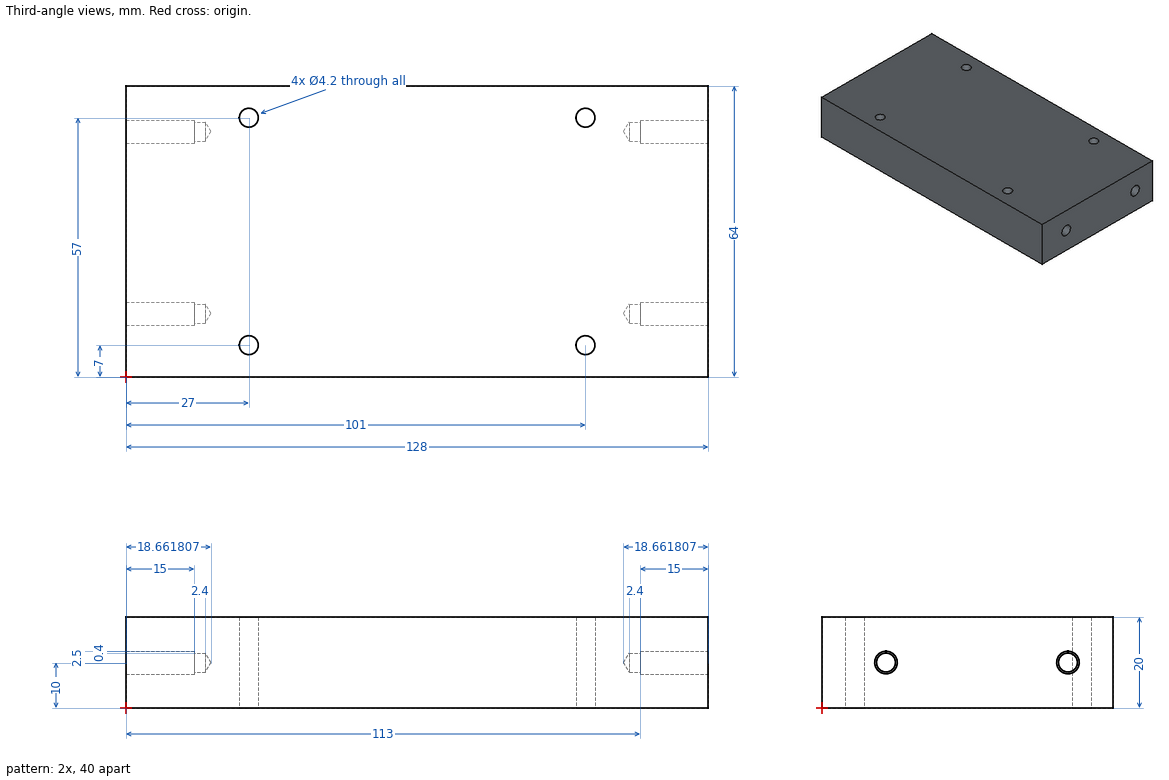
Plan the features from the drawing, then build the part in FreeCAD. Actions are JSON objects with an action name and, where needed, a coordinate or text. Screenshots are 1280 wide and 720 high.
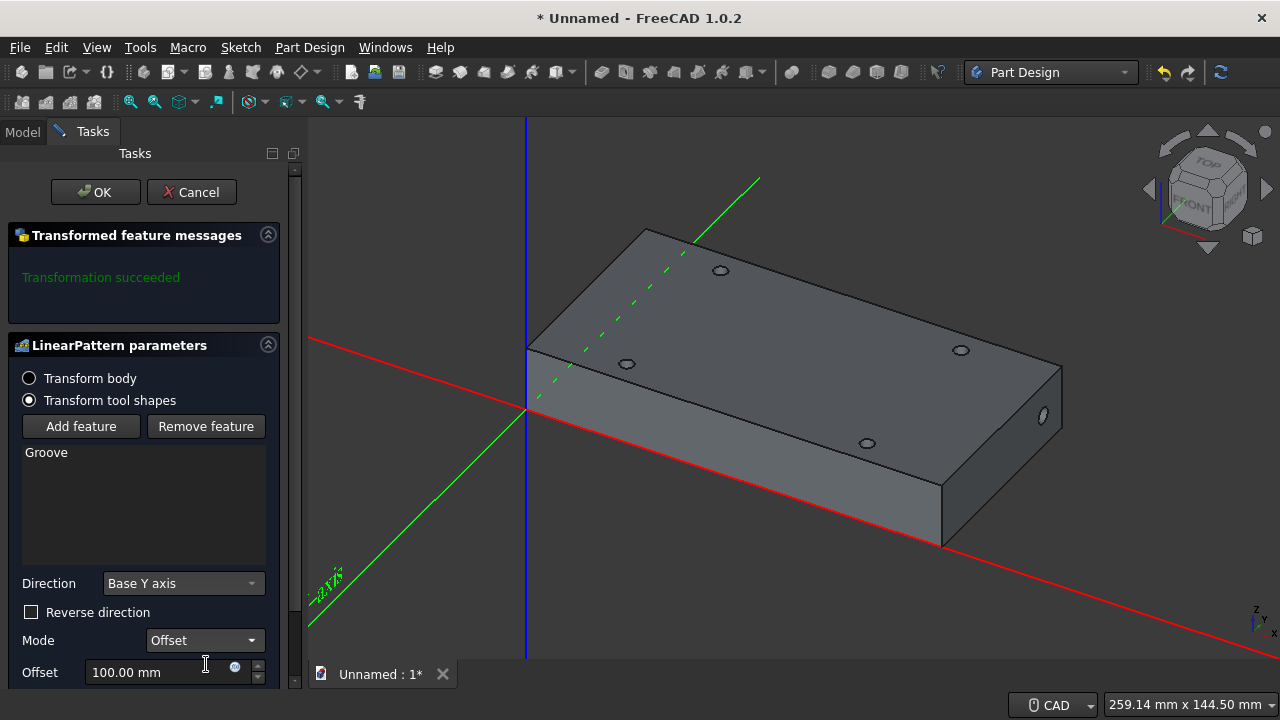
{"action": "triple_click", "coordinate": [168, 672]}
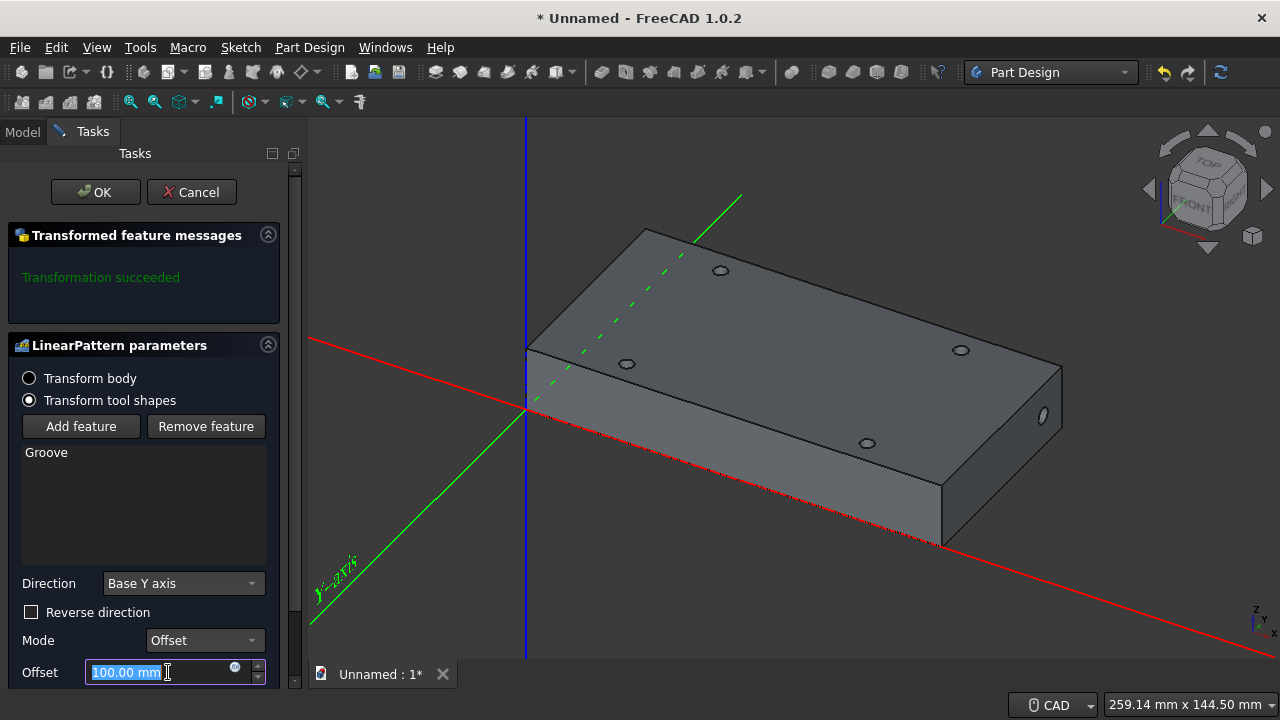
{"action": "type", "text": "40"}
{"action": "key", "text": "Tab"}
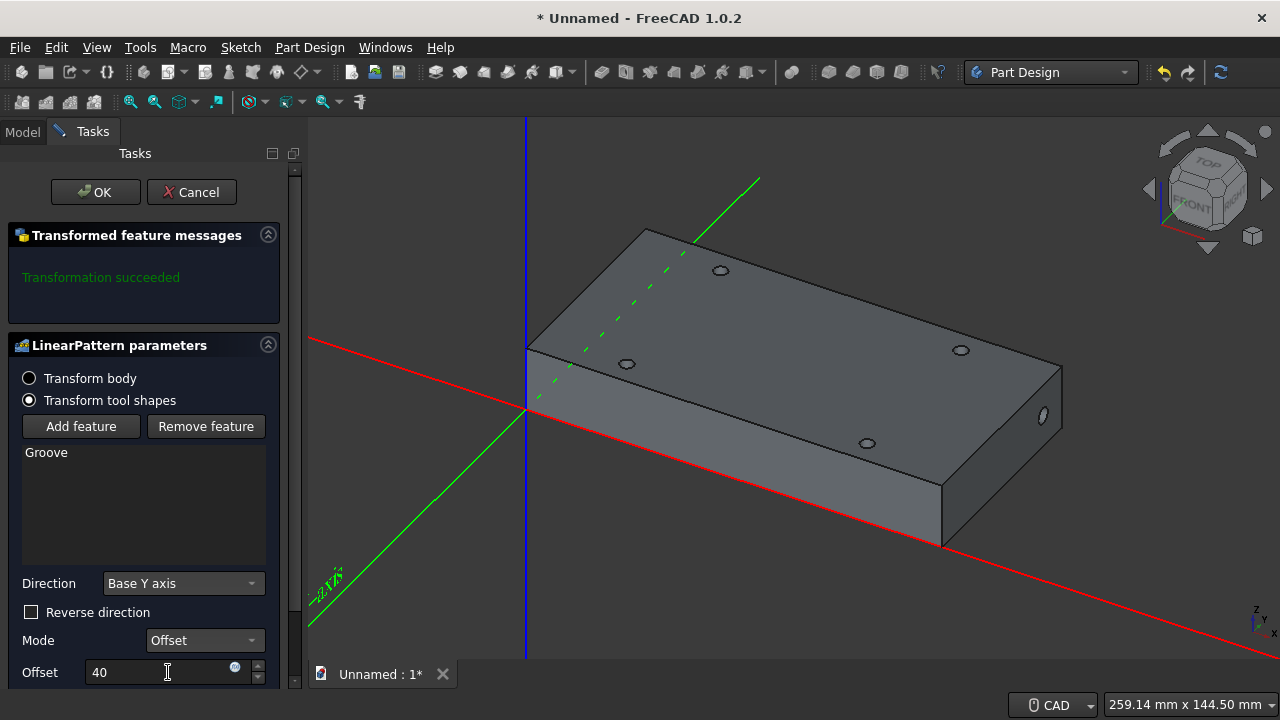
{"action": "scroll", "coordinate": [295, 426], "scroll_direction": "down", "scroll_amount": 2}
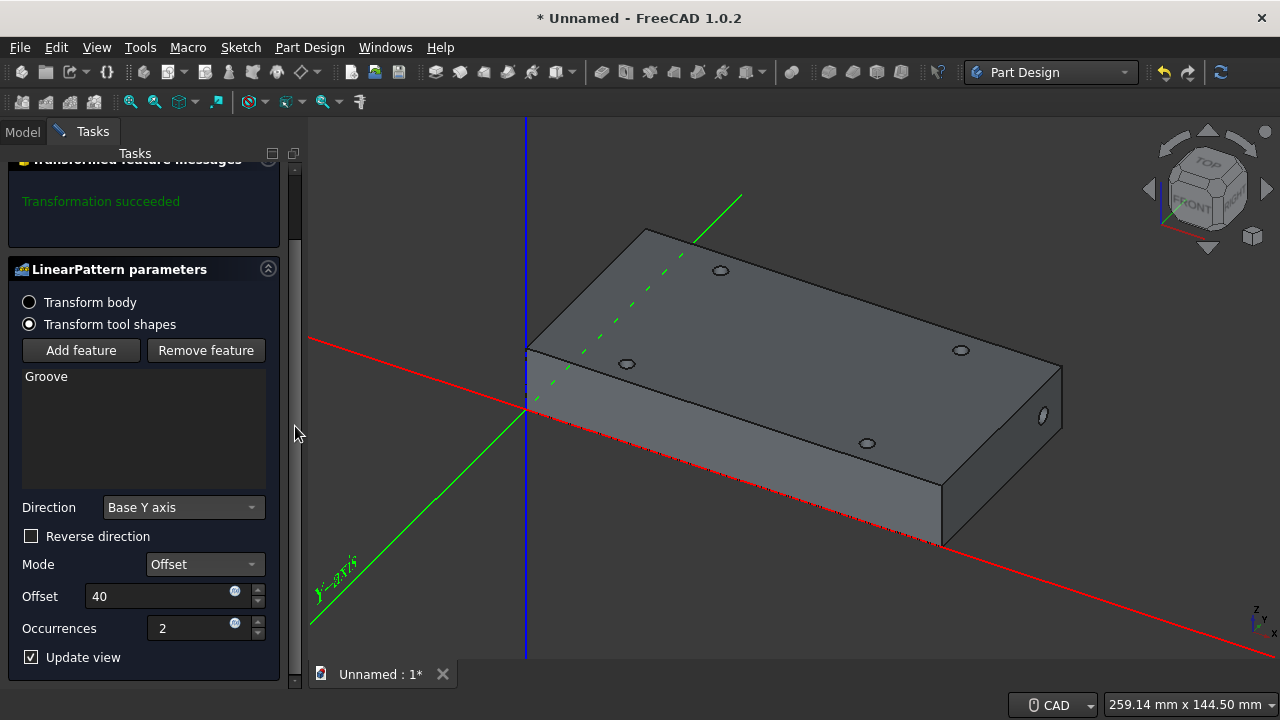
{"action": "triple_click", "coordinate": [198, 628]}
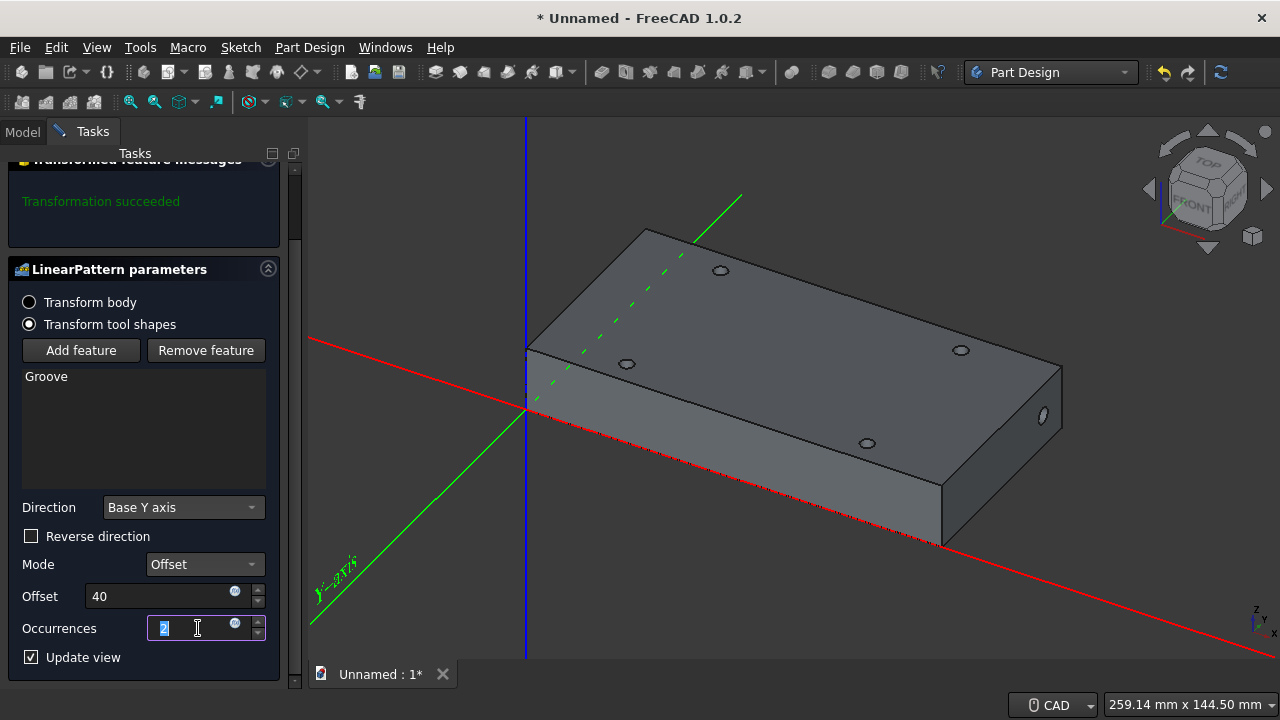
{"action": "type", "text": "2"}
{"action": "key", "text": "Tab"}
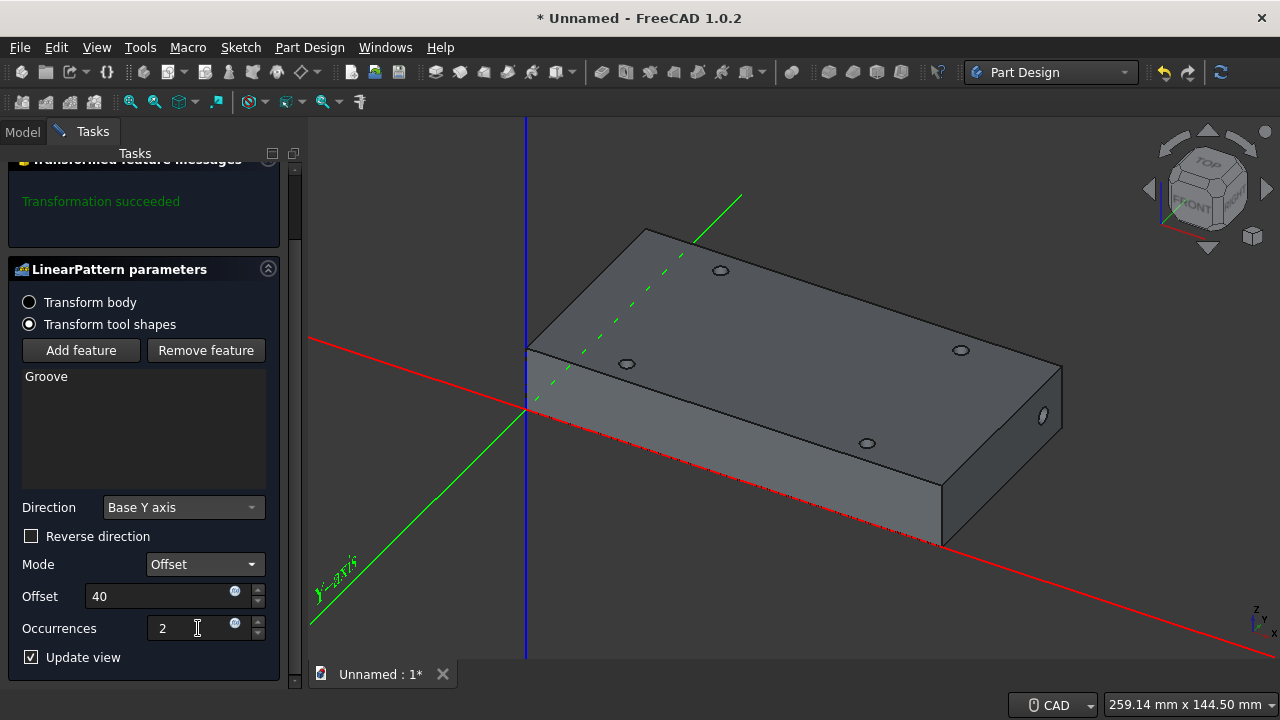
{"action": "left_click", "coordinate": [30, 536]}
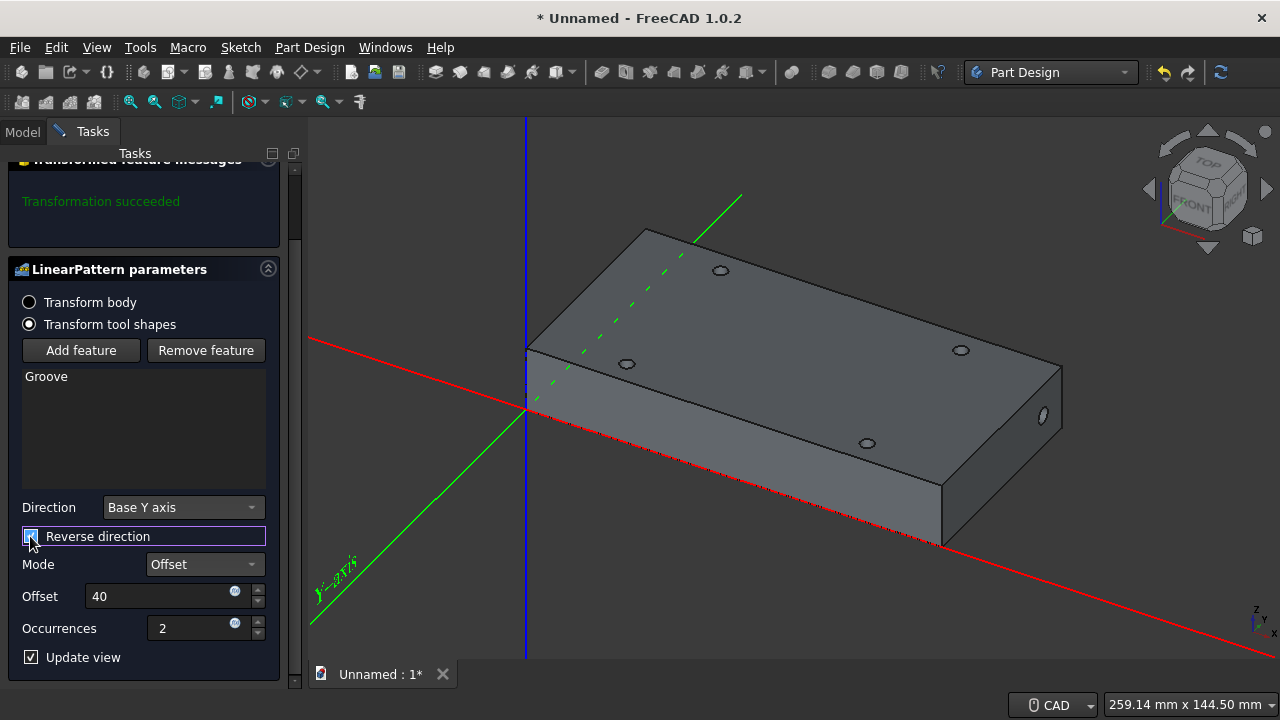
{"action": "scroll", "coordinate": [295, 426], "scroll_direction": "up", "scroll_amount": 3}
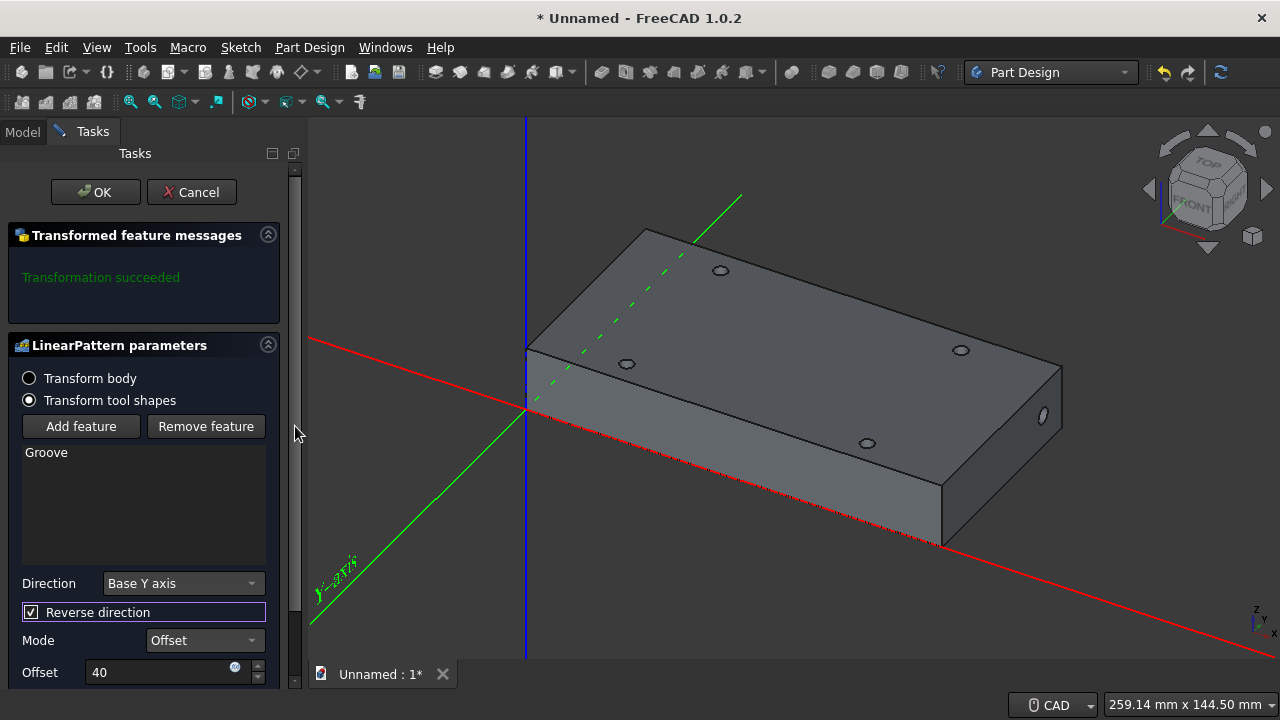
{"action": "left_click", "coordinate": [96, 192]}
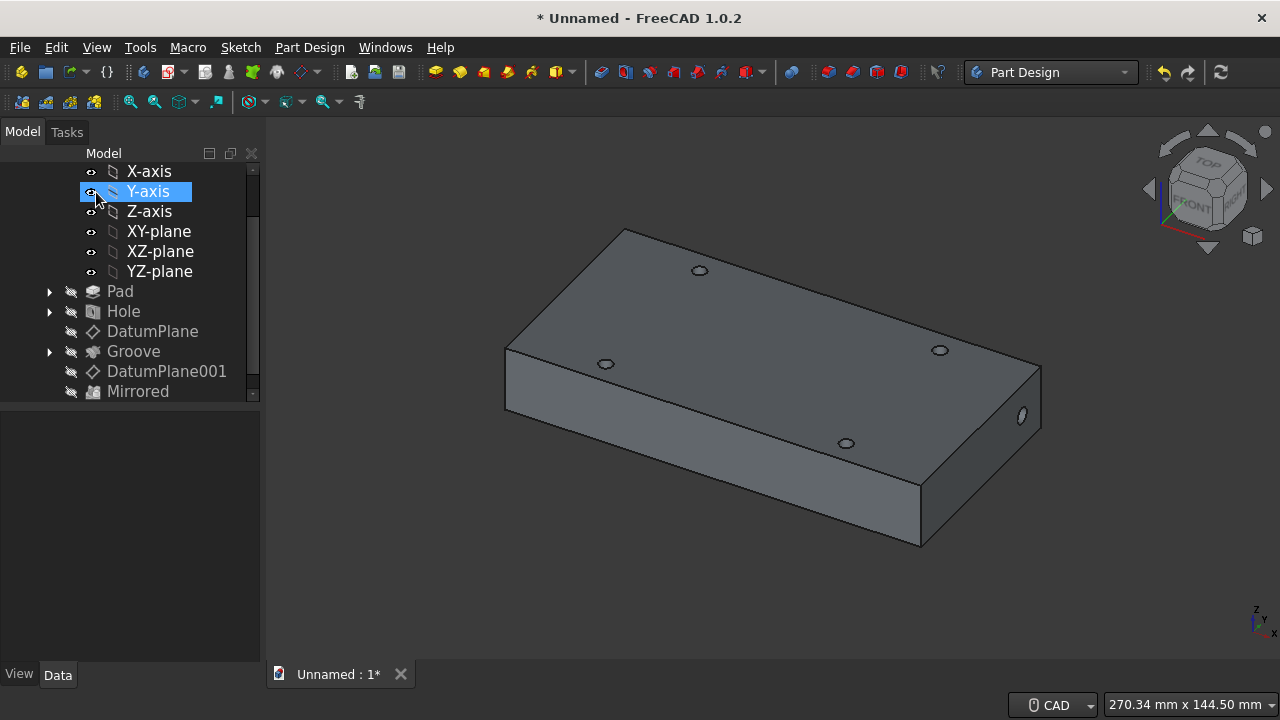
{"action": "scroll", "coordinate": [160, 287], "scroll_direction": "down", "scroll_amount": 3}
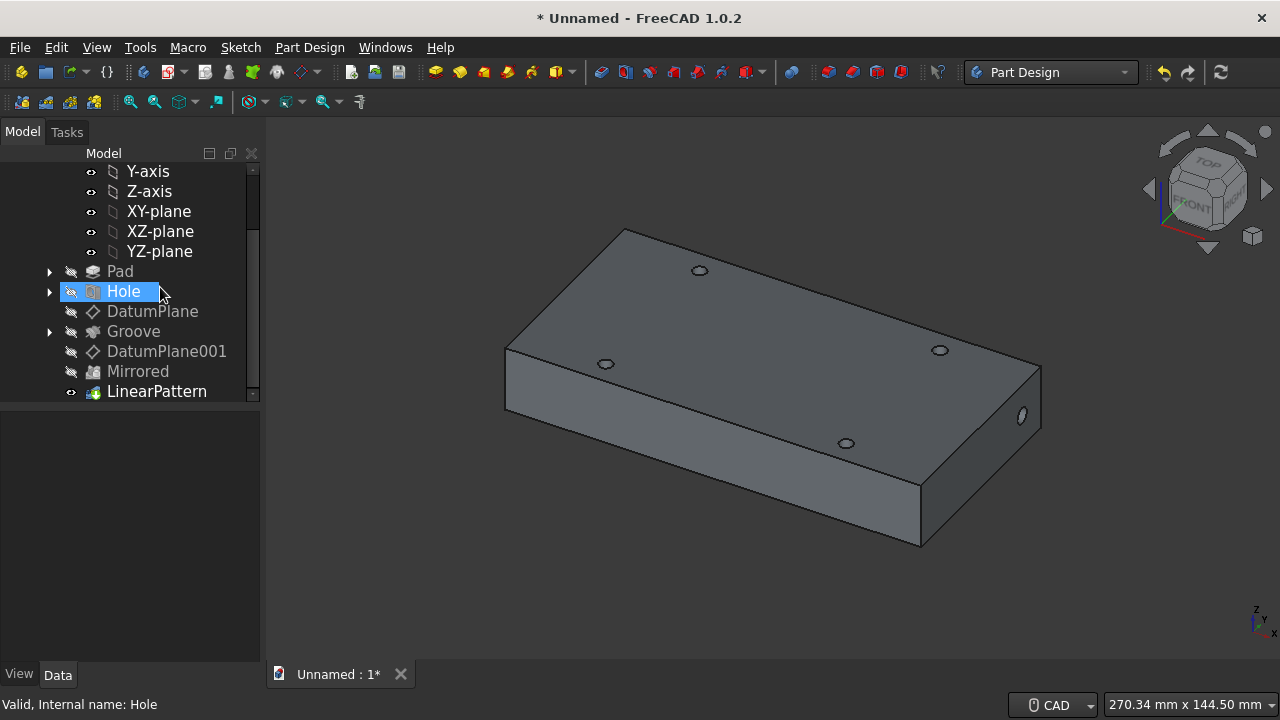
{"action": "scroll", "coordinate": [160, 287], "scroll_direction": "up", "scroll_amount": 15}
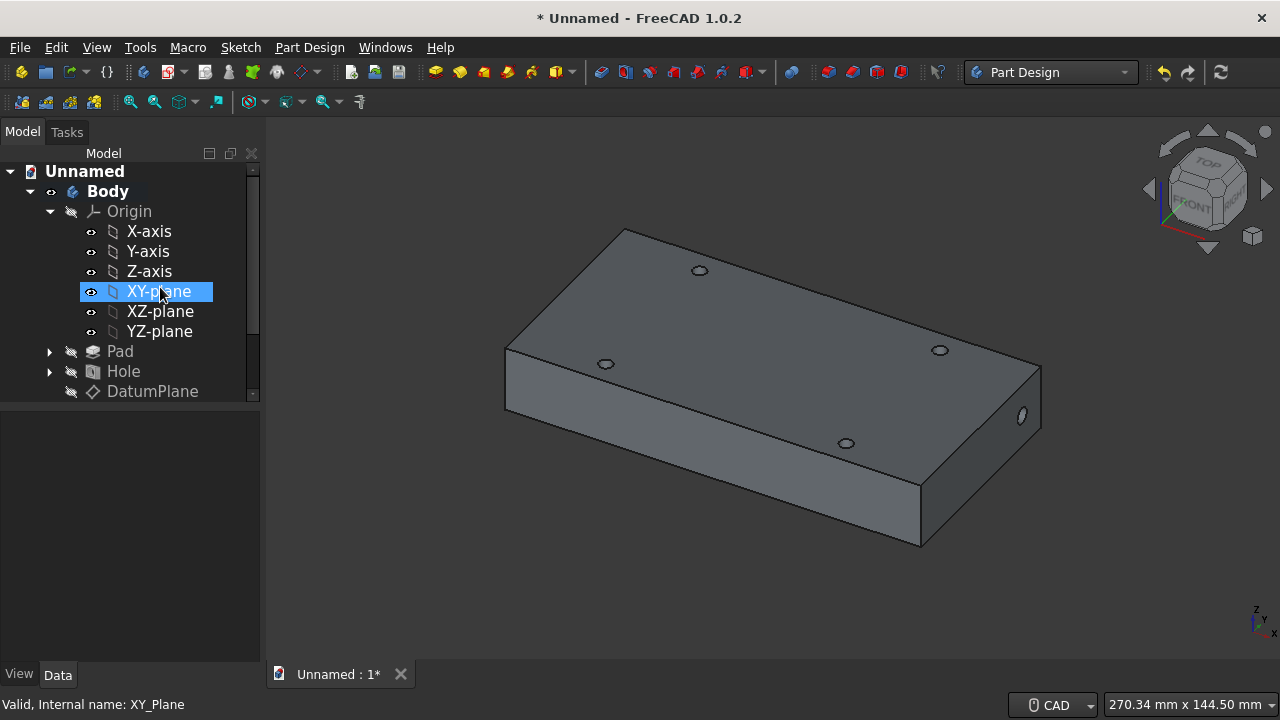
{"action": "left_click", "coordinate": [136, 312]}